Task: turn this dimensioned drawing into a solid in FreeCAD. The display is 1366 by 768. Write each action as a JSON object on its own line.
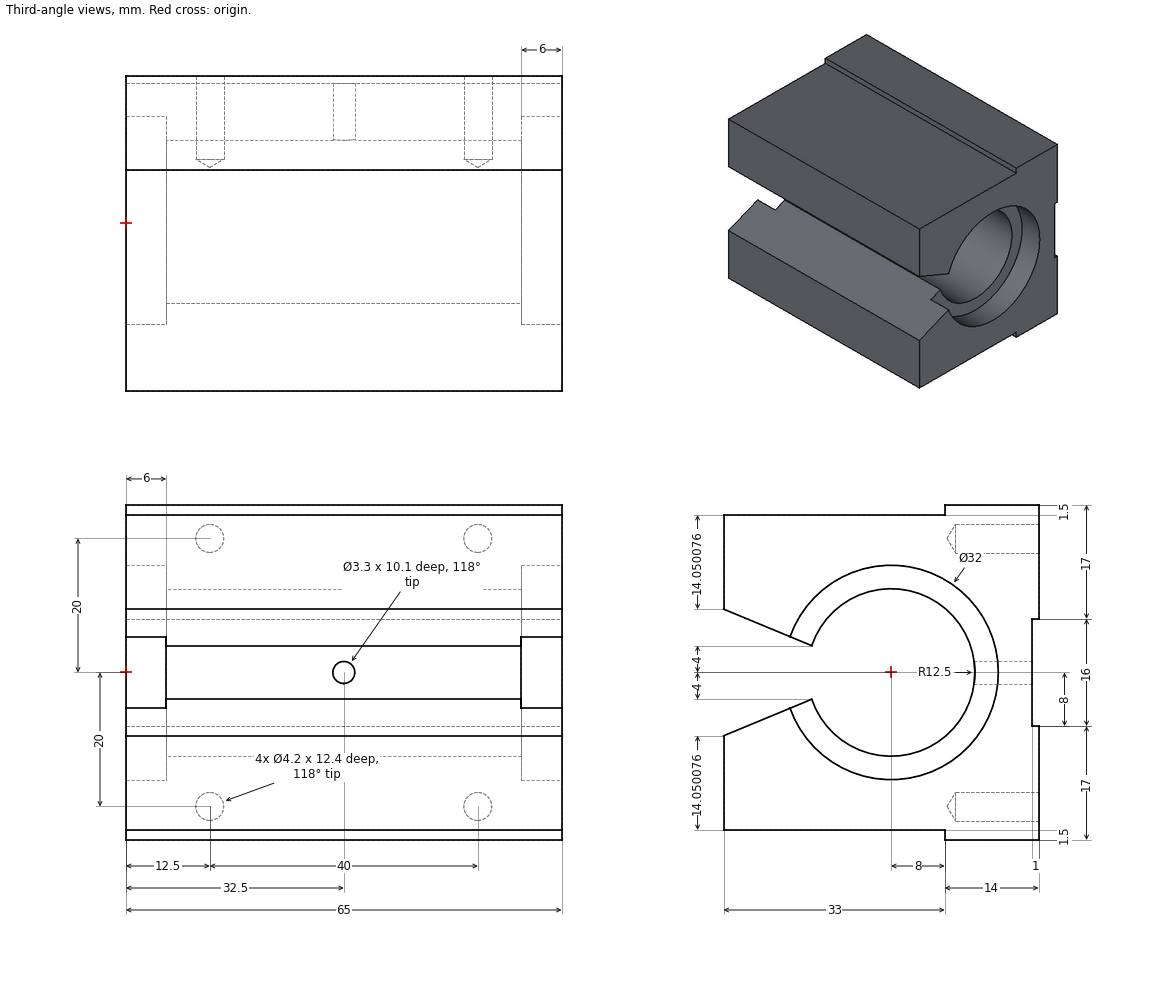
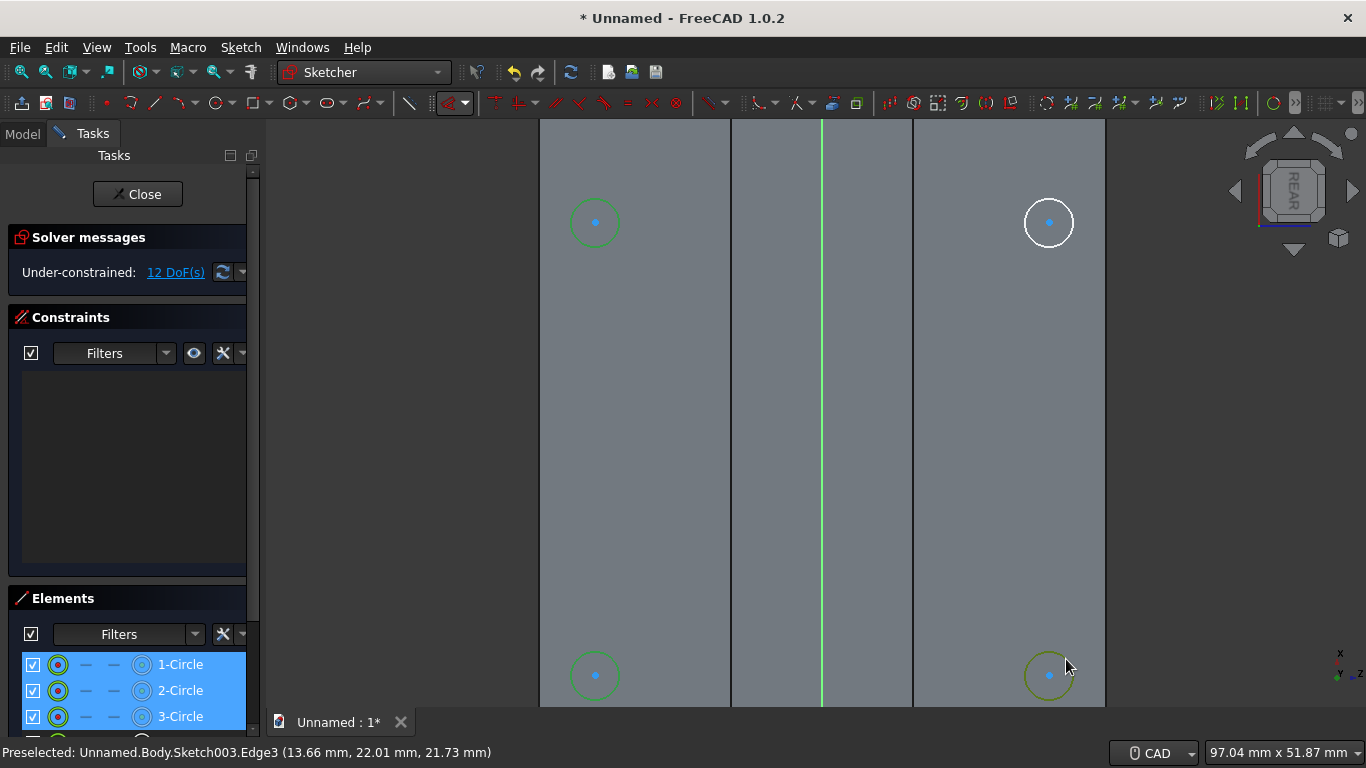
{"action": "left_click", "coordinate": [1066, 206]}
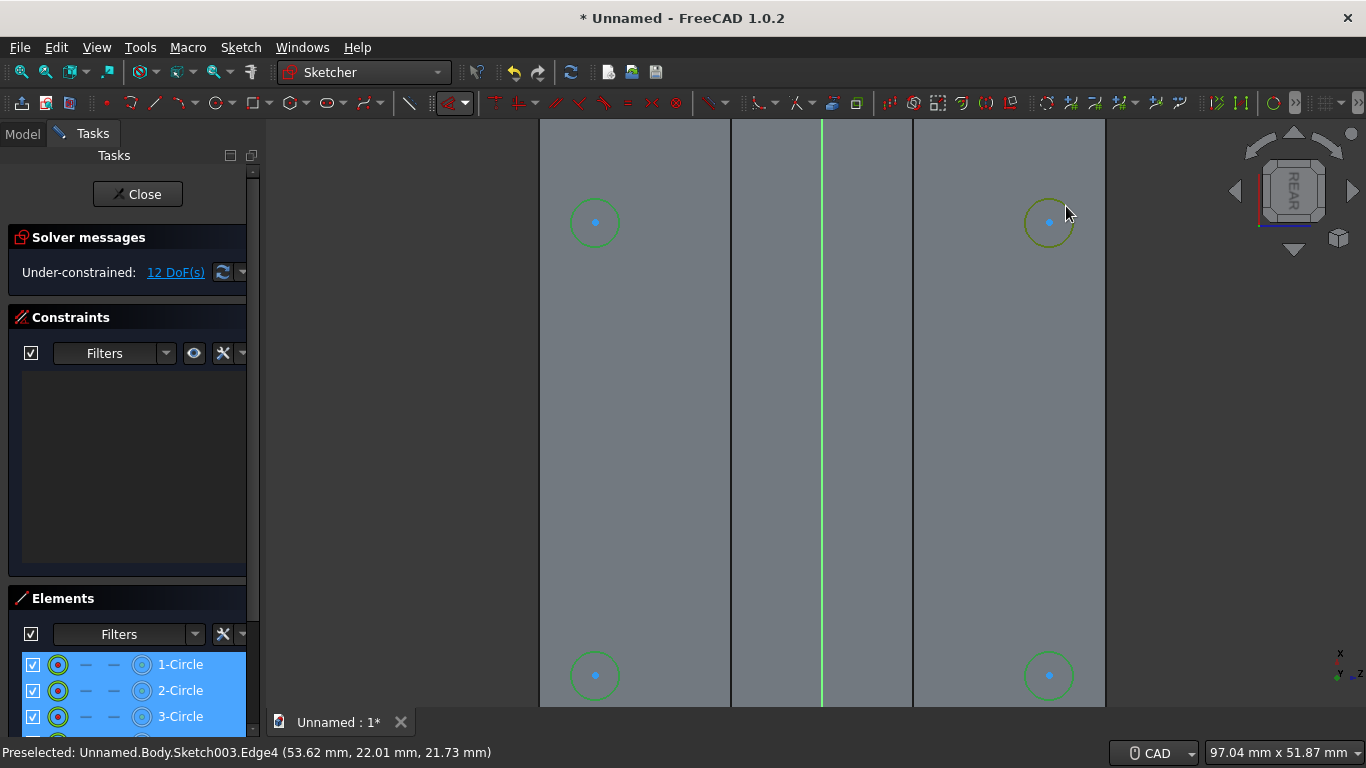
{"action": "left_click", "coordinate": [628, 104]}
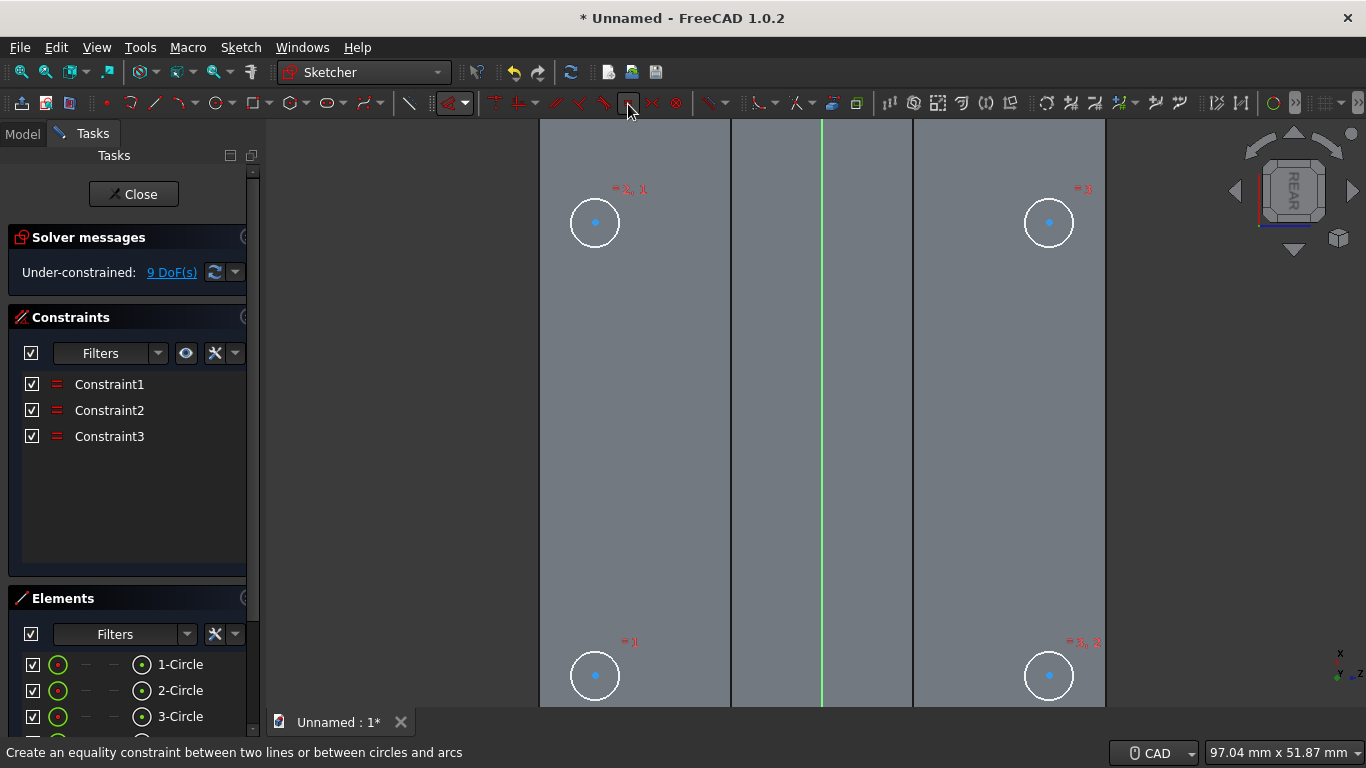
{"action": "left_click", "coordinate": [595, 676]}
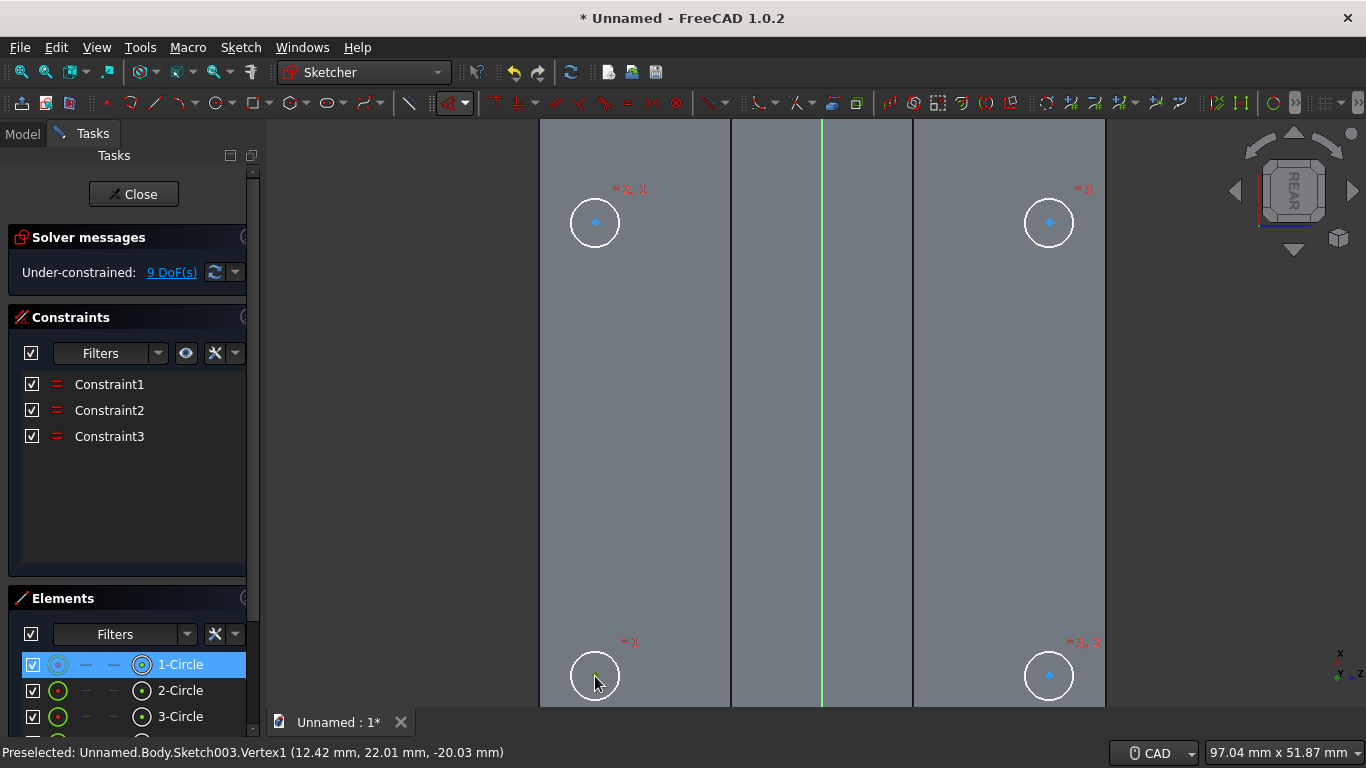
{"action": "left_click", "coordinate": [595, 223]}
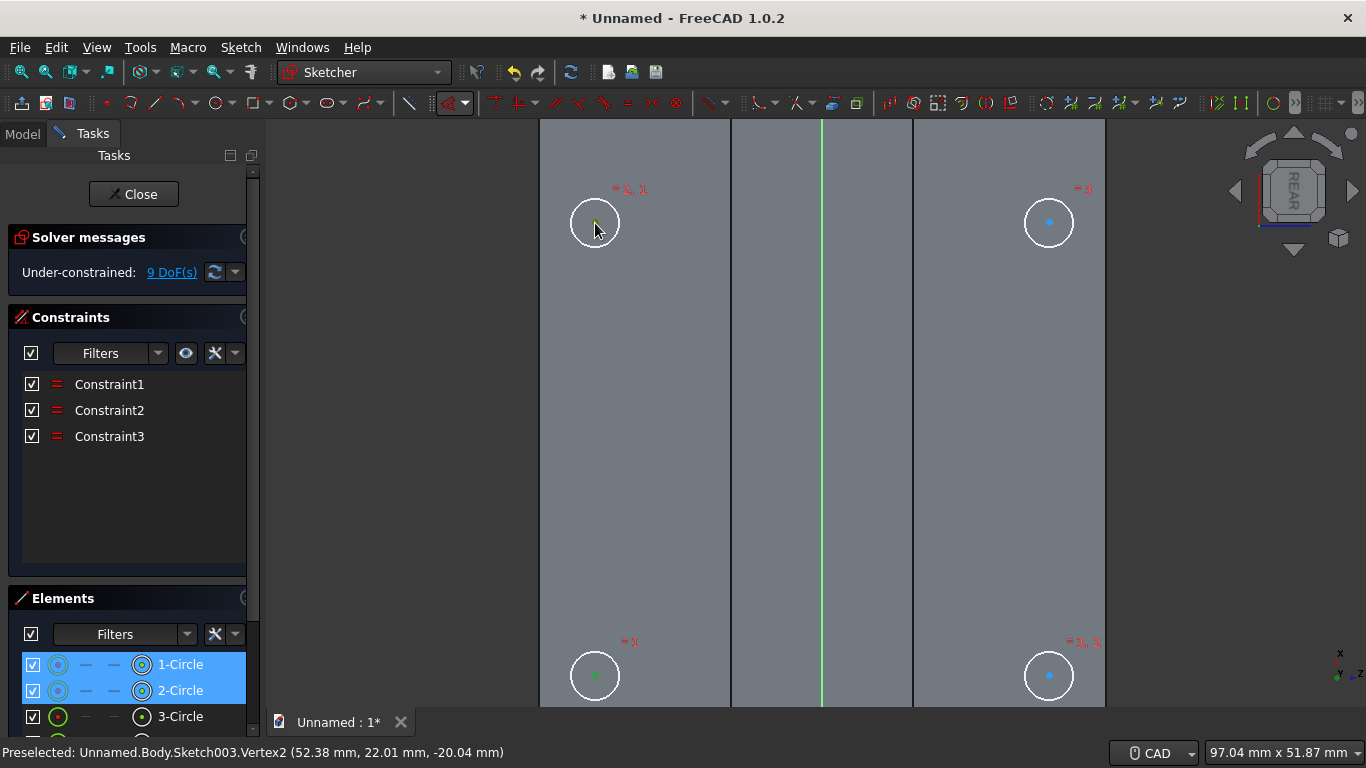
{"action": "key", "text": "v"}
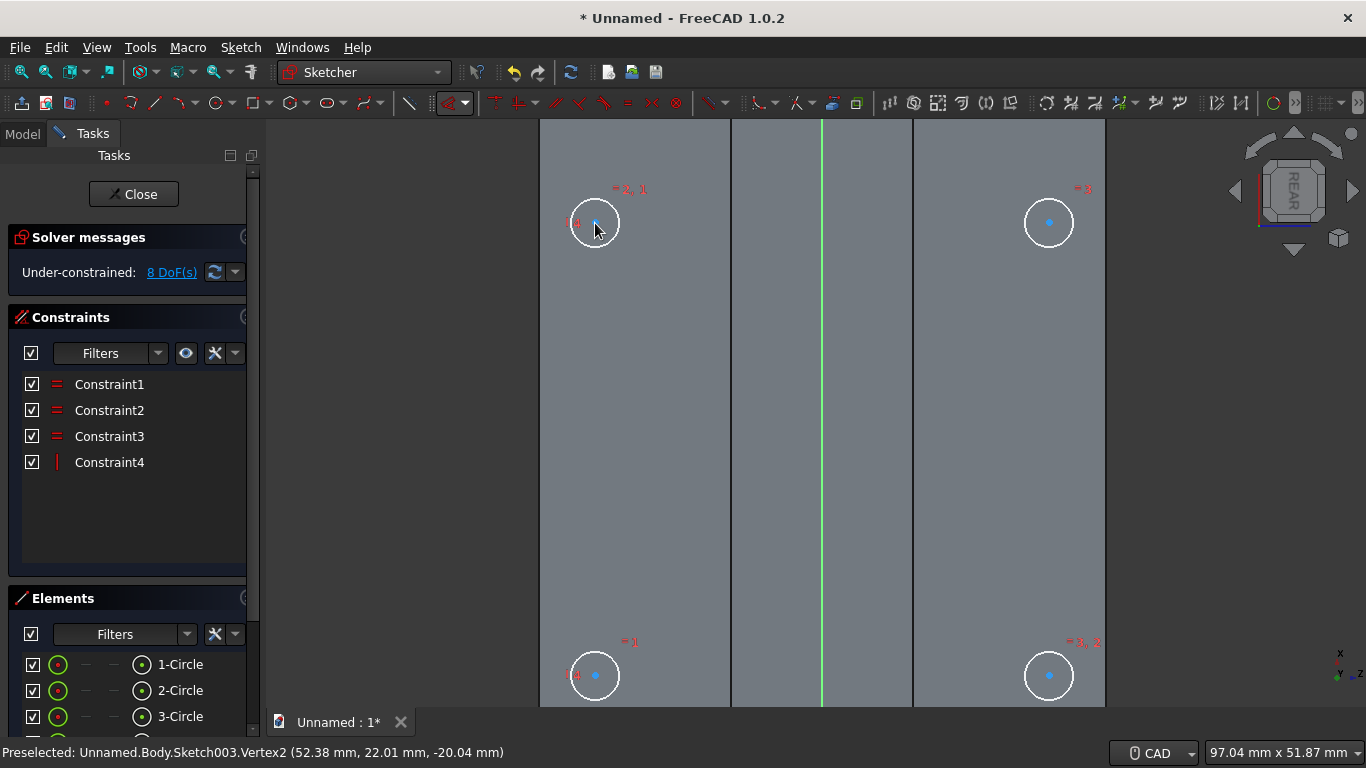
{"action": "left_click", "coordinate": [595, 676]}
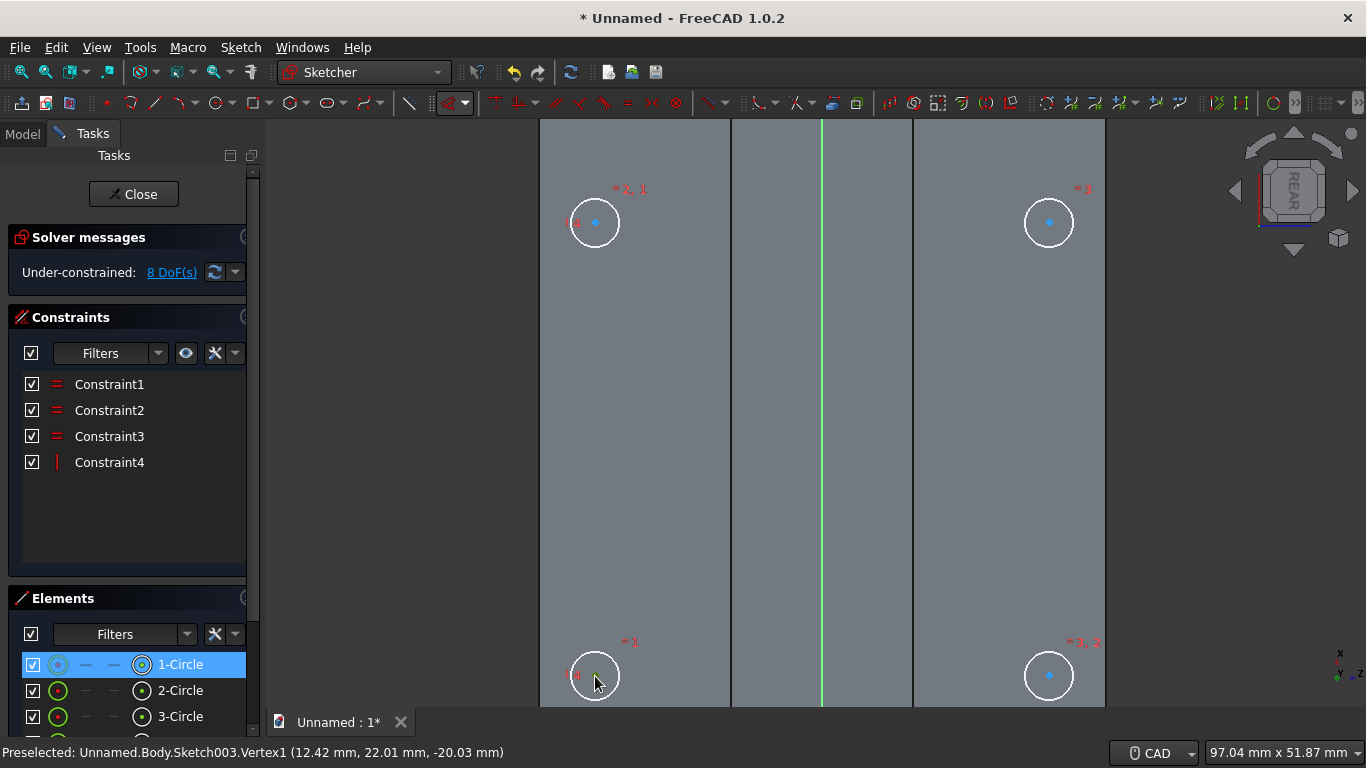
{"action": "left_click", "coordinate": [1049, 676]}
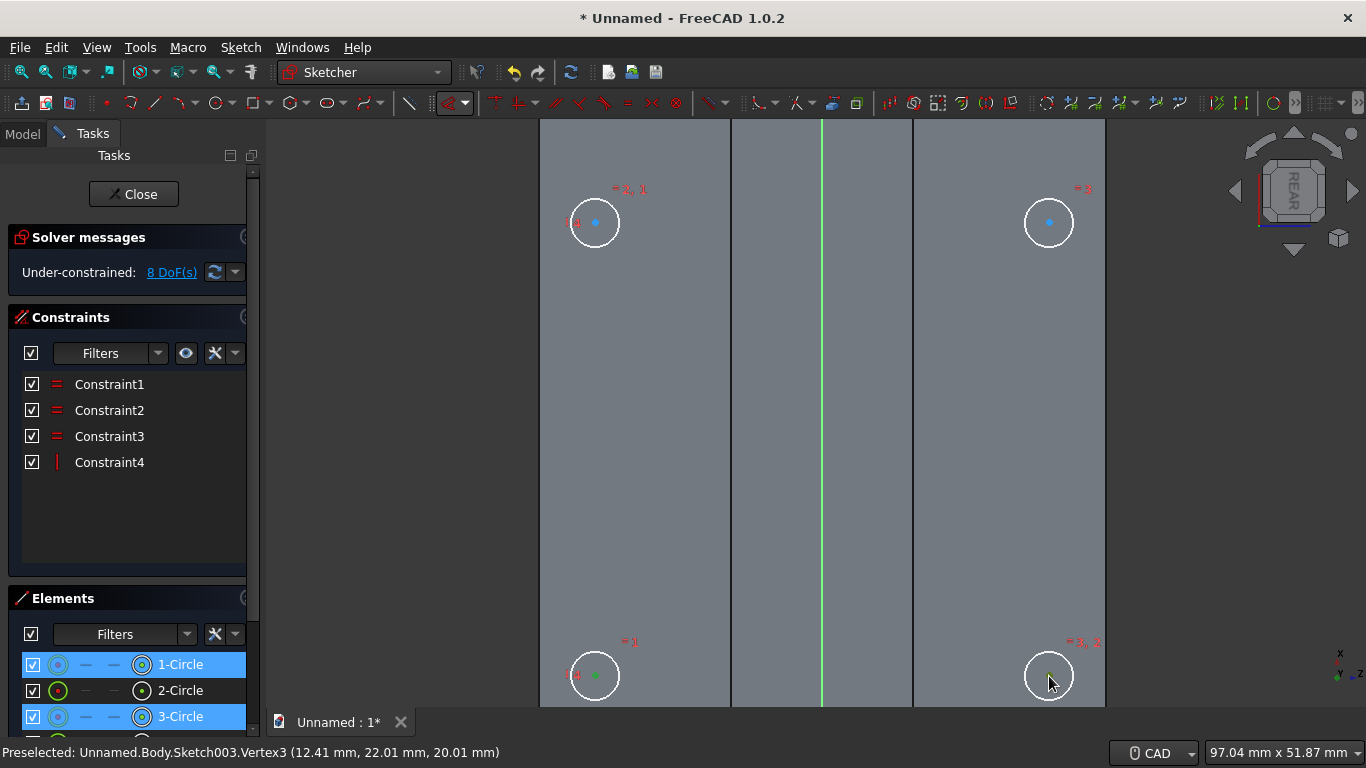
{"action": "key", "text": "h"}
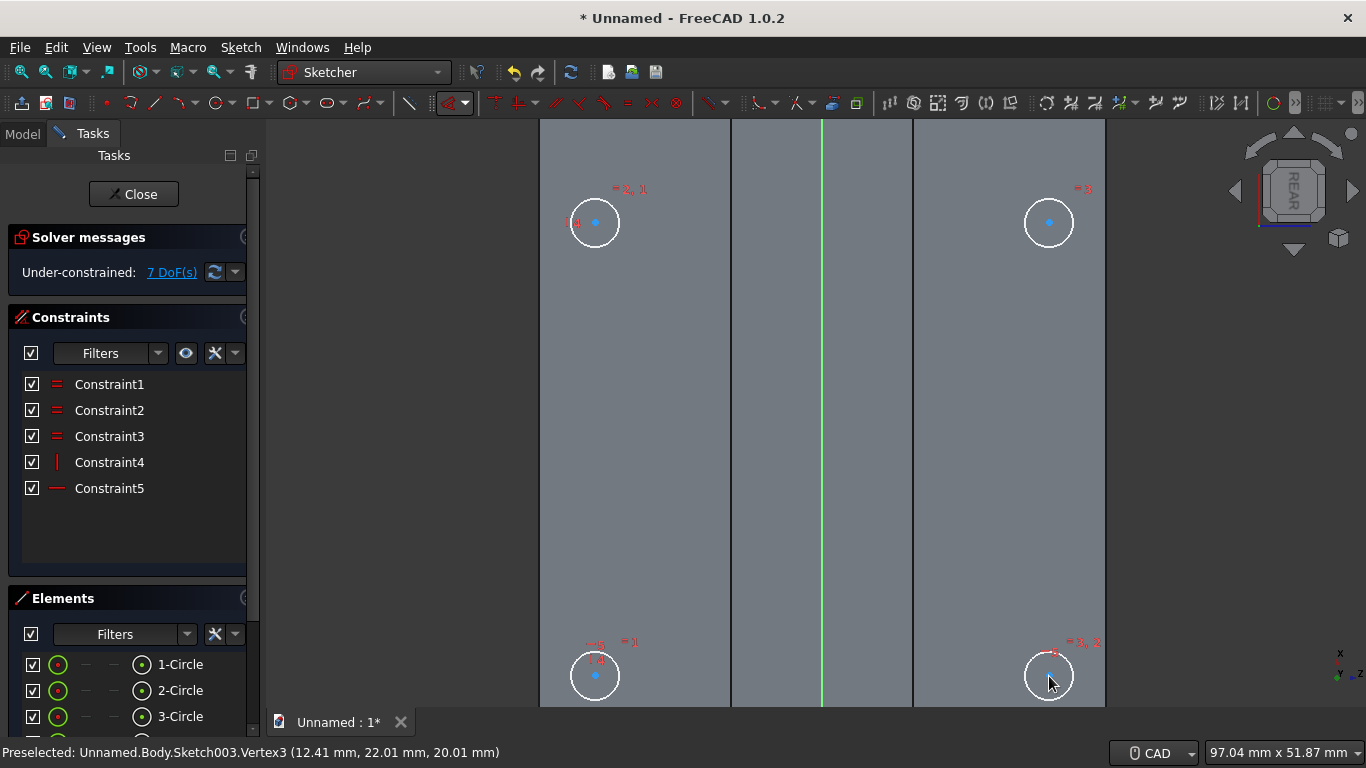
{"action": "left_click", "coordinate": [1049, 676]}